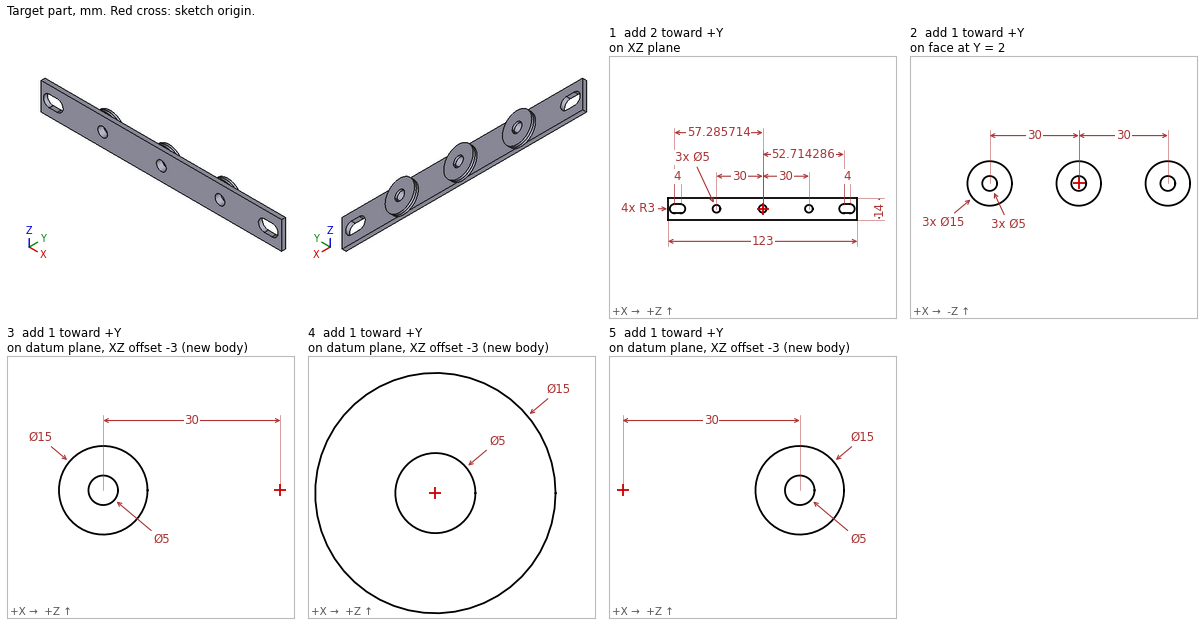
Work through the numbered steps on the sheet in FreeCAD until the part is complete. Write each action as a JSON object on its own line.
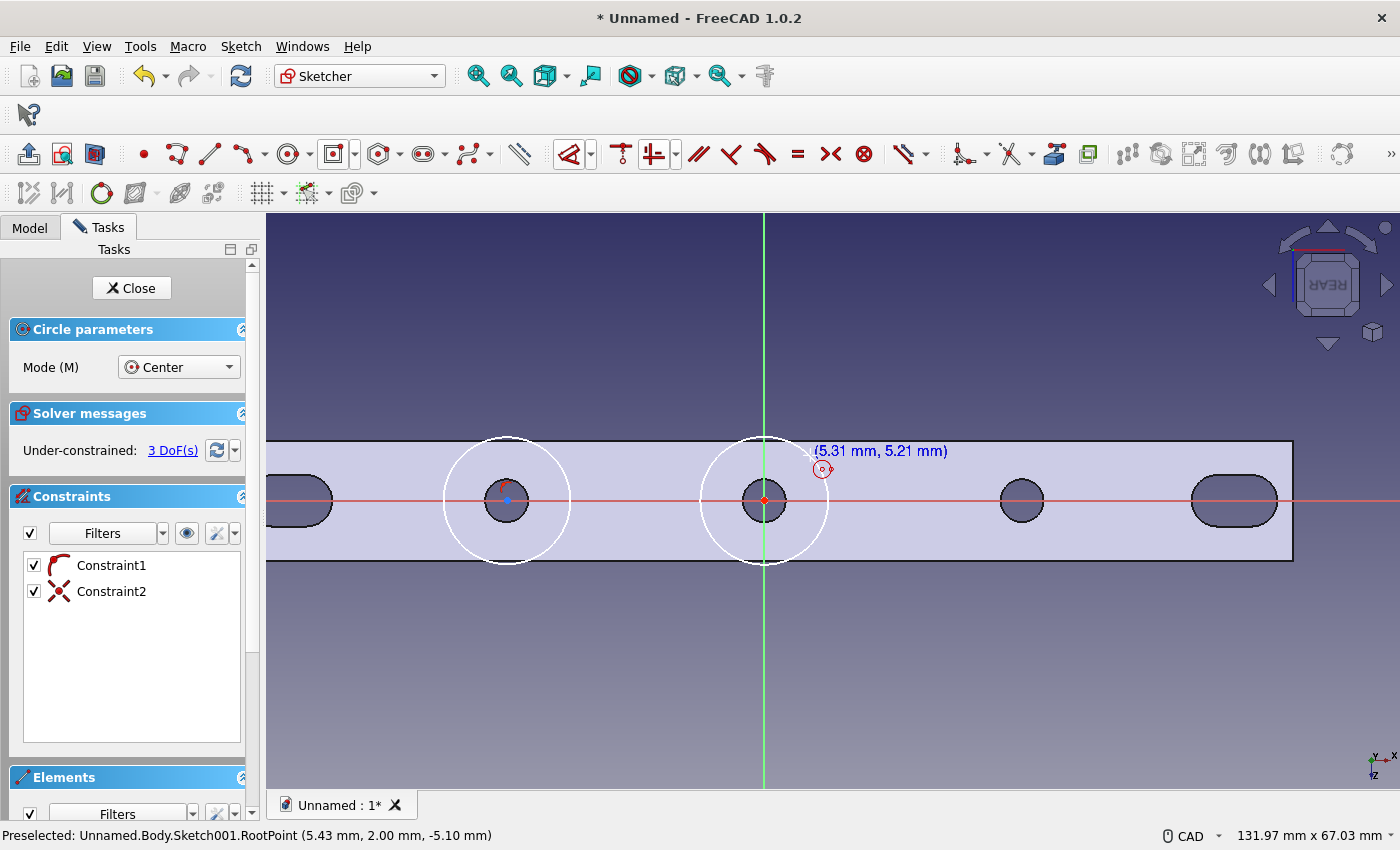
{"action": "left_click", "coordinate": [1022, 501]}
{"action": "left_click", "coordinate": [1068, 455]}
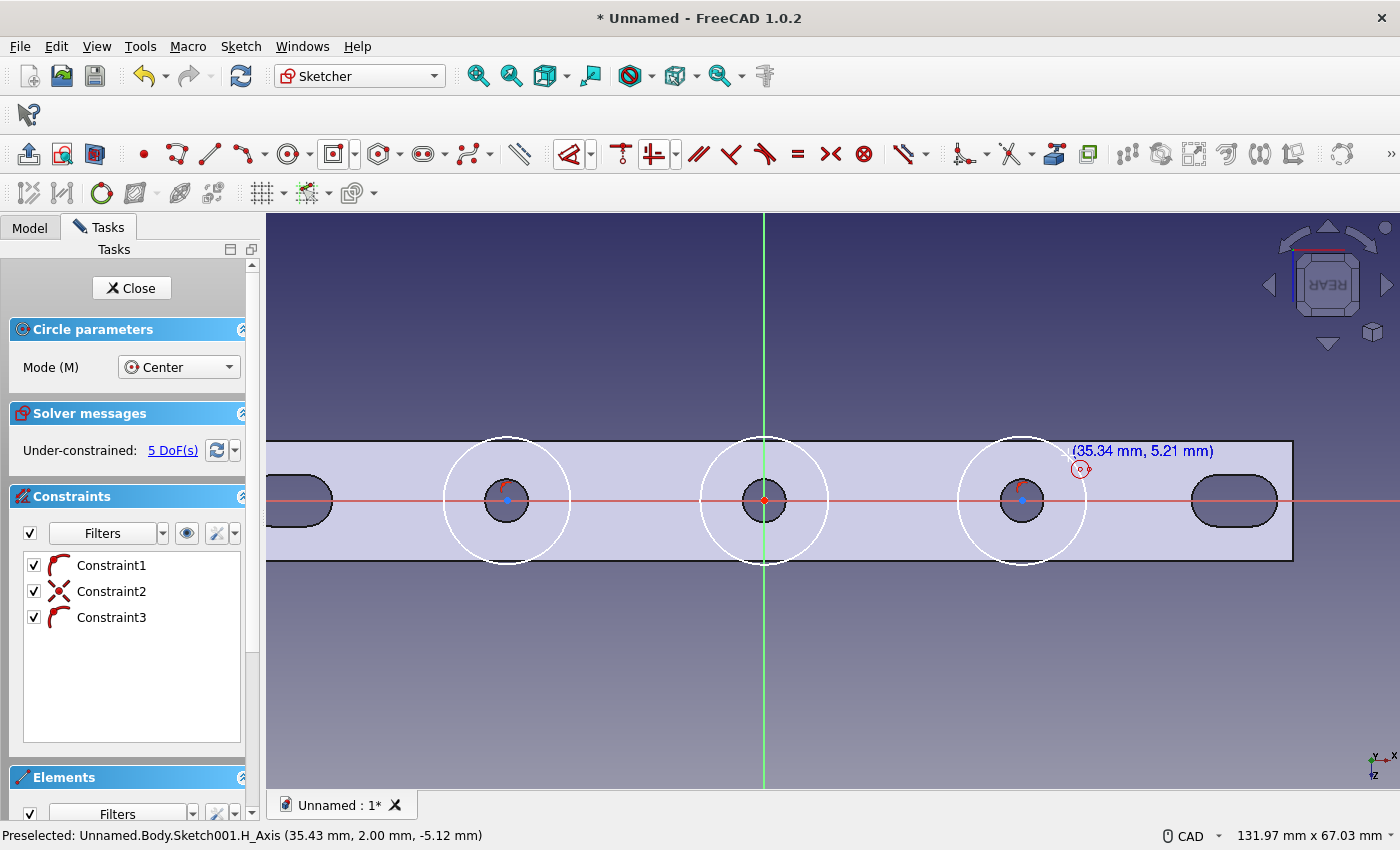
{"action": "left_click", "coordinate": [507, 501]}
{"action": "left_click", "coordinate": [522, 486]}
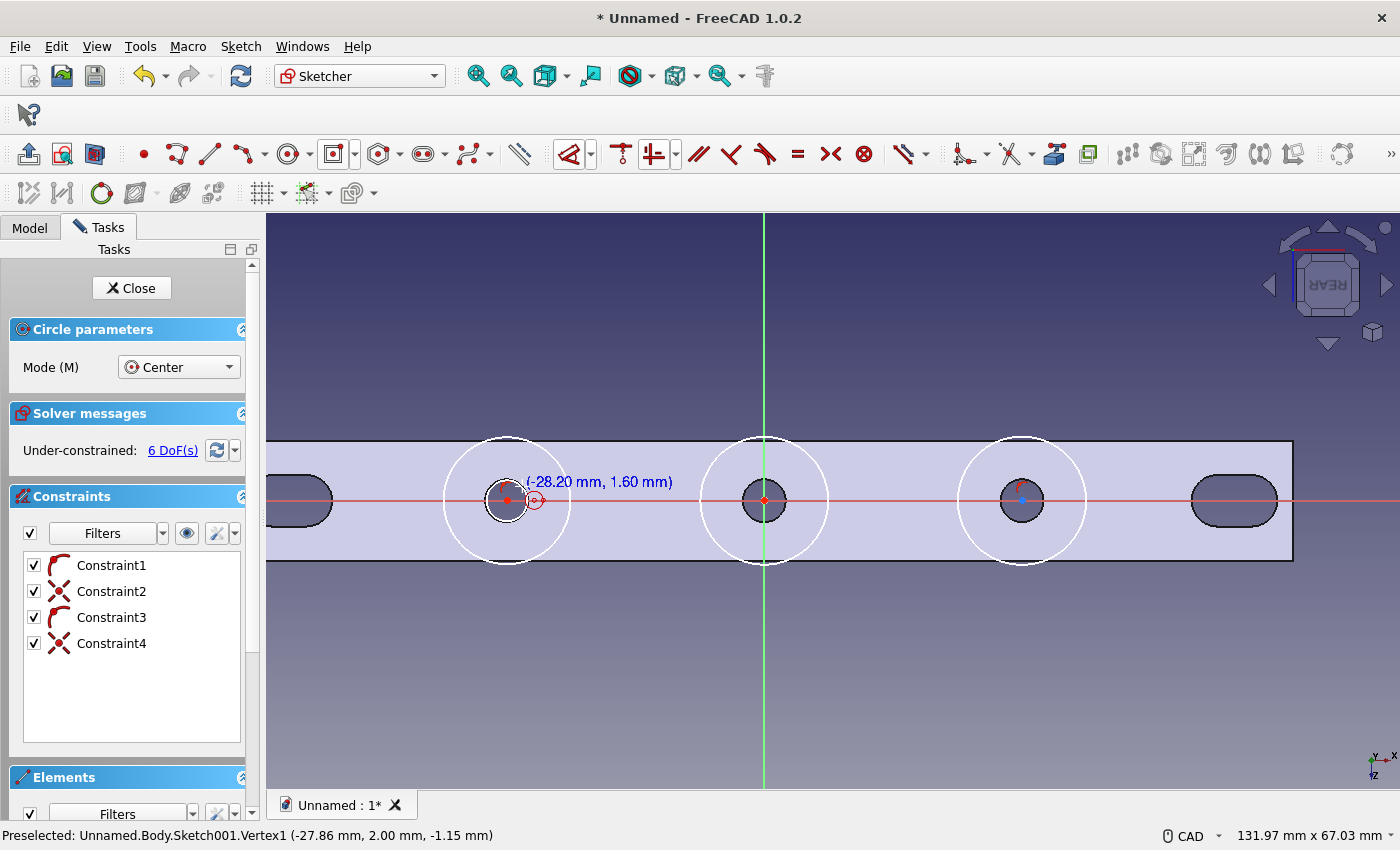
{"action": "left_click", "coordinate": [764, 501]}
{"action": "left_click", "coordinate": [780, 486]}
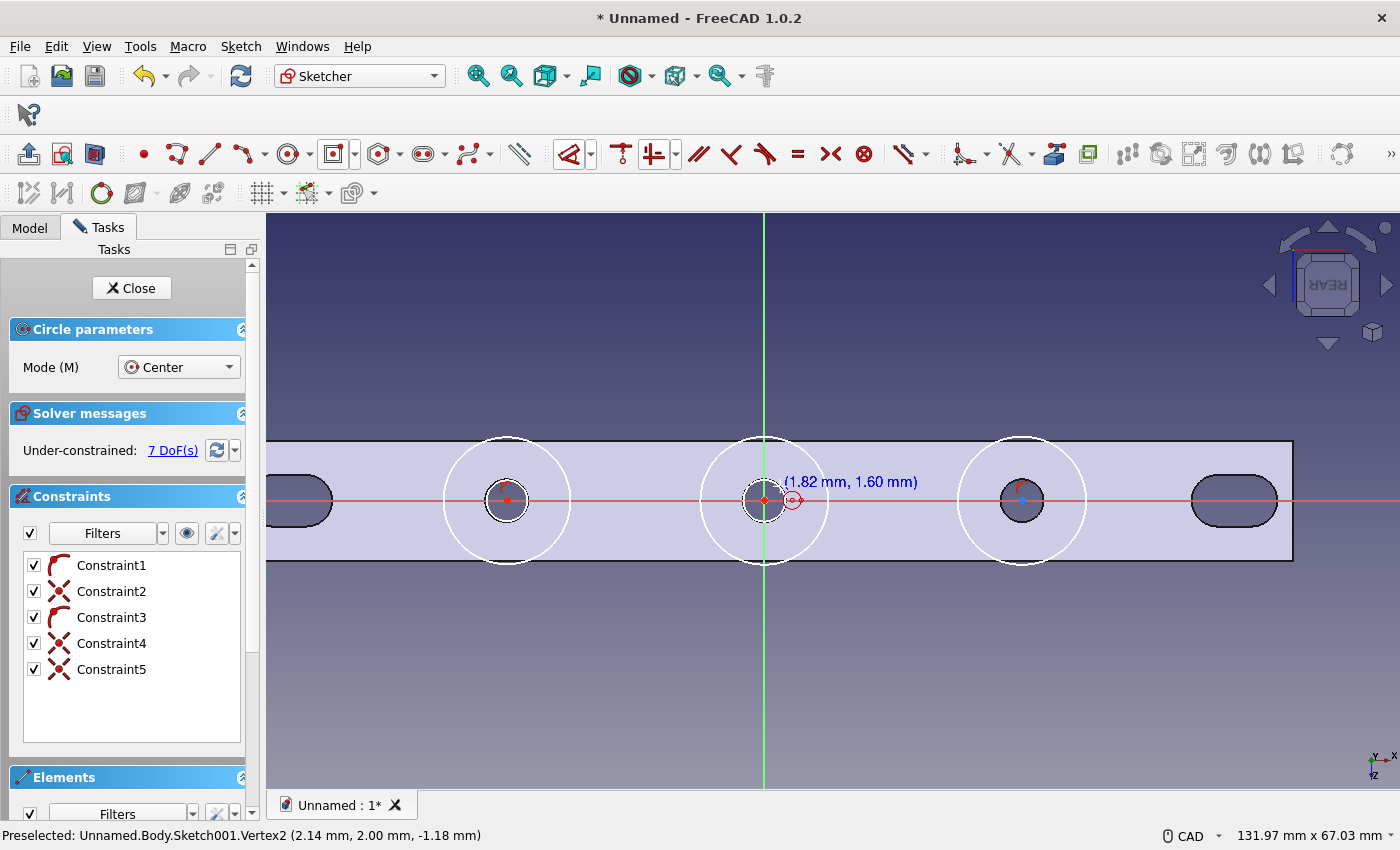
{"action": "left_click", "coordinate": [1022, 501]}
{"action": "left_click", "coordinate": [1037, 486]}
{"action": "key", "text": "Escape"}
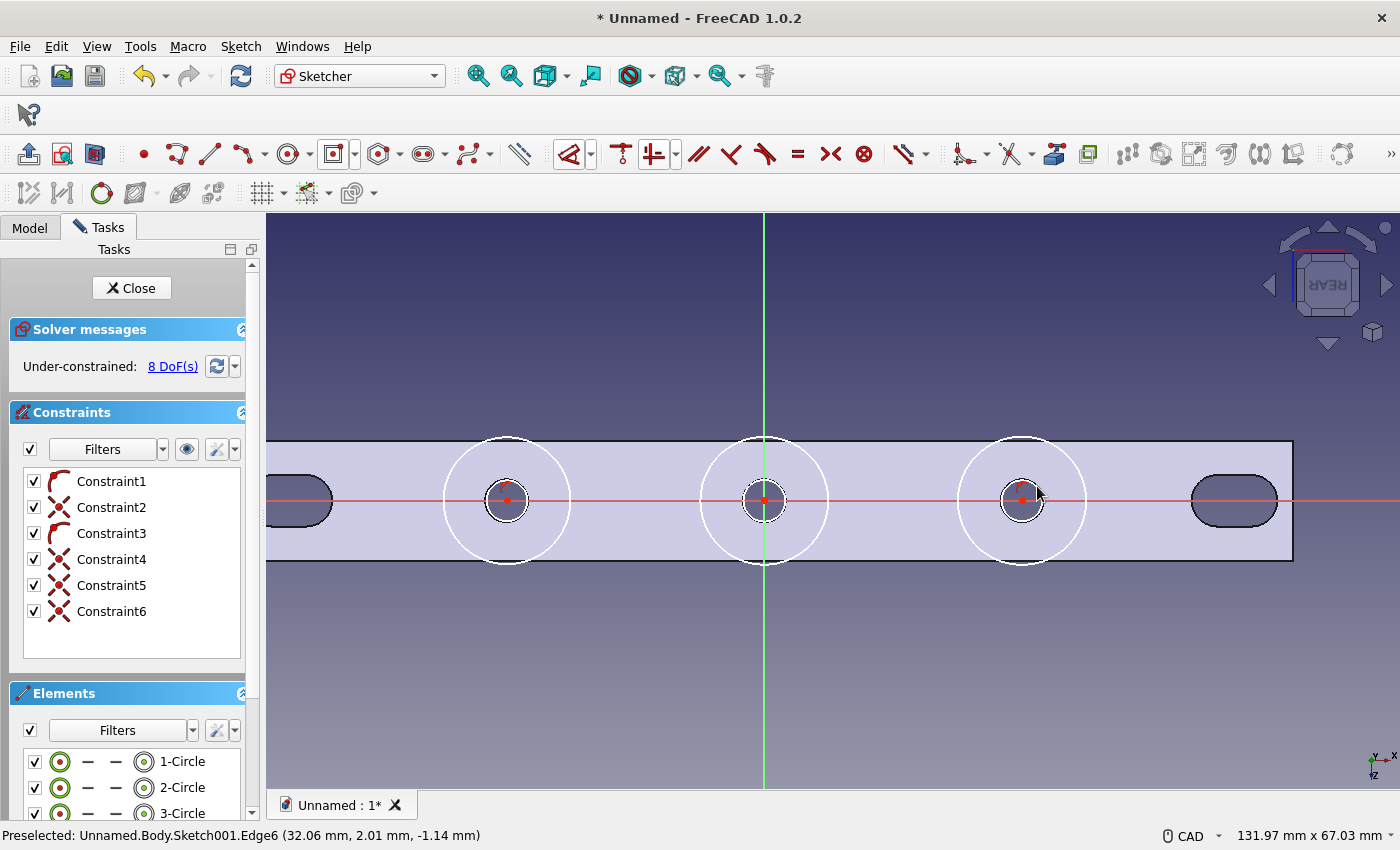
{"action": "left_click", "coordinate": [552, 456]}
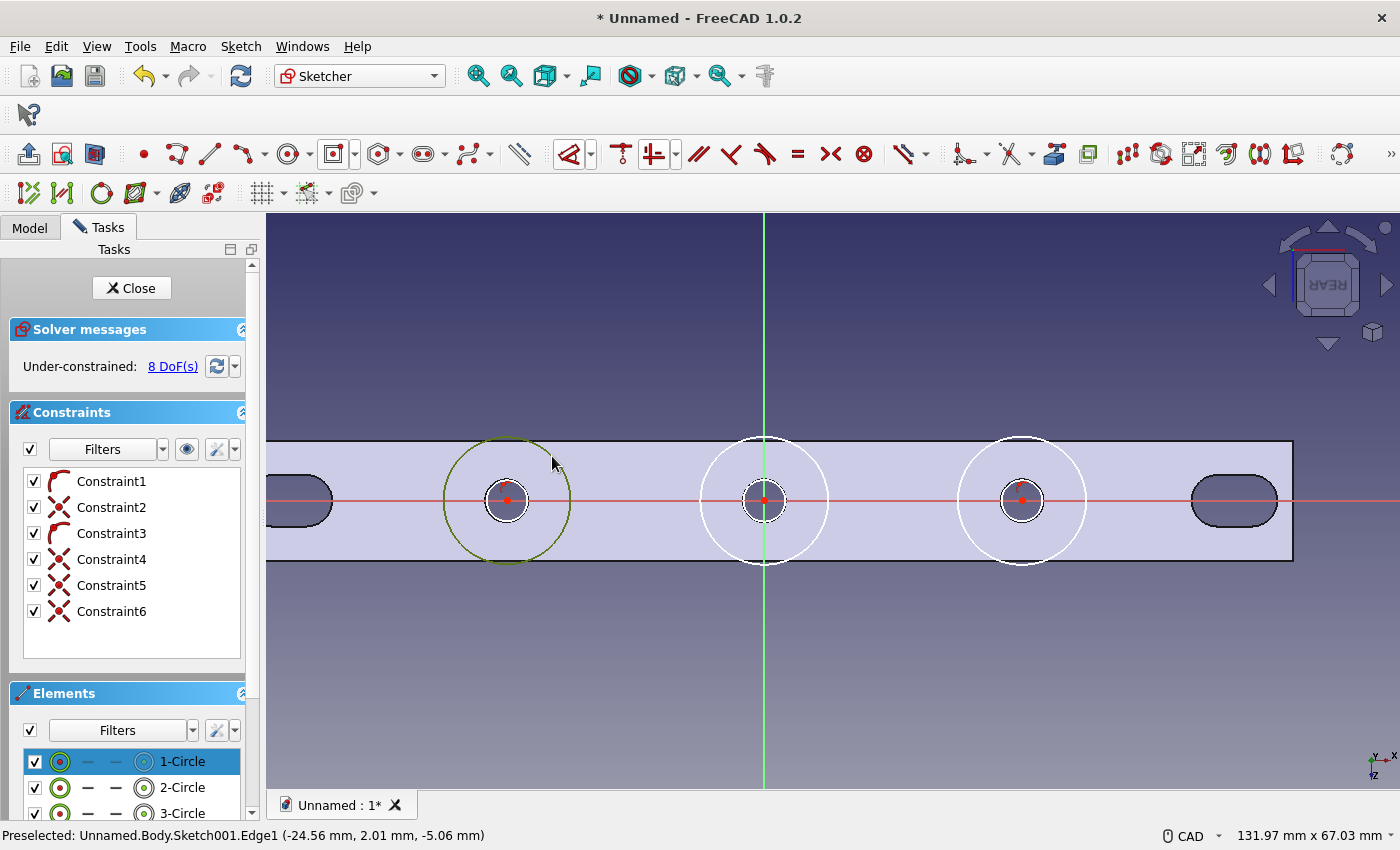
{"action": "left_click", "coordinate": [809, 455]}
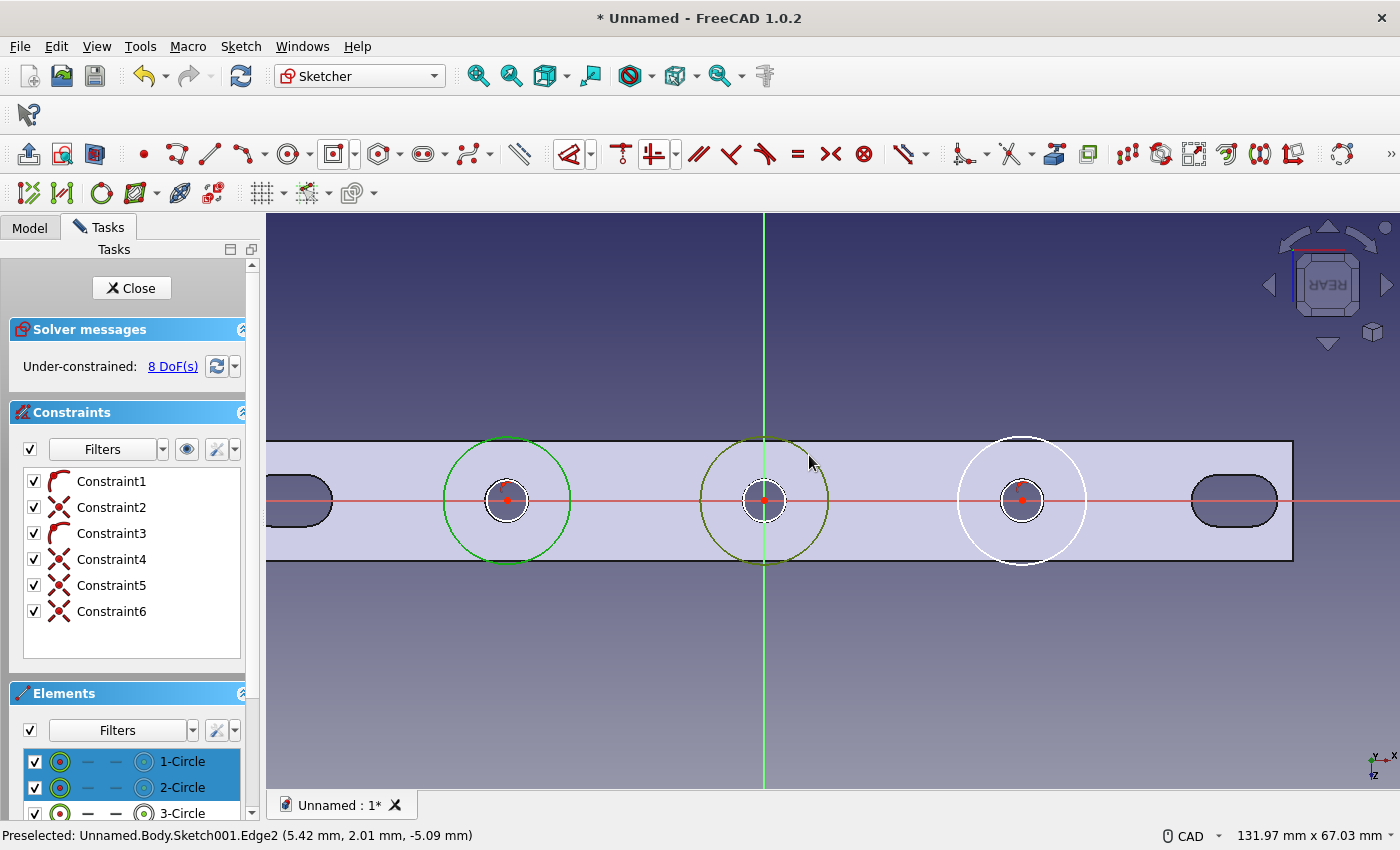
{"action": "left_click", "coordinate": [1067, 455]}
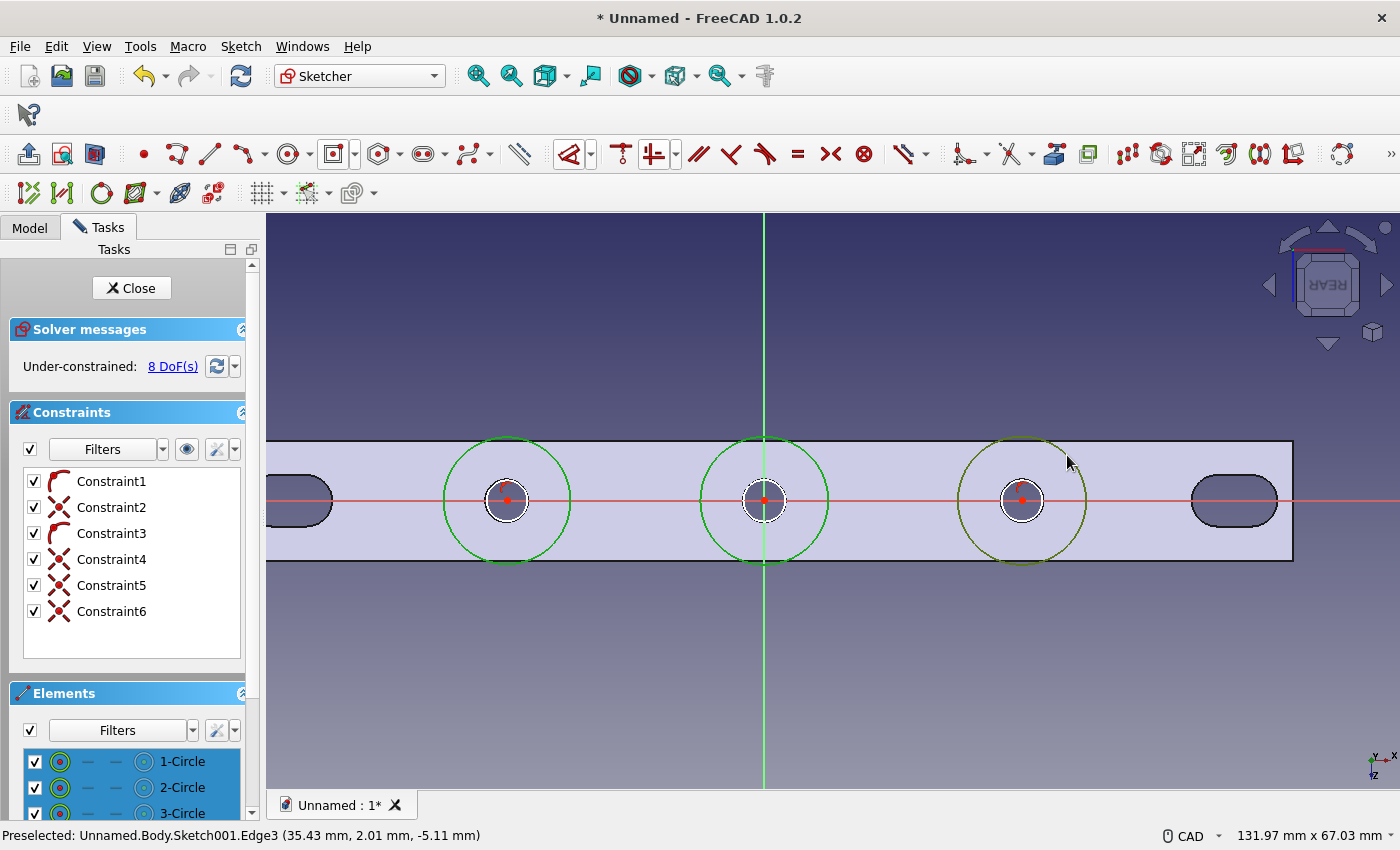
{"action": "left_click", "coordinate": [798, 154]}